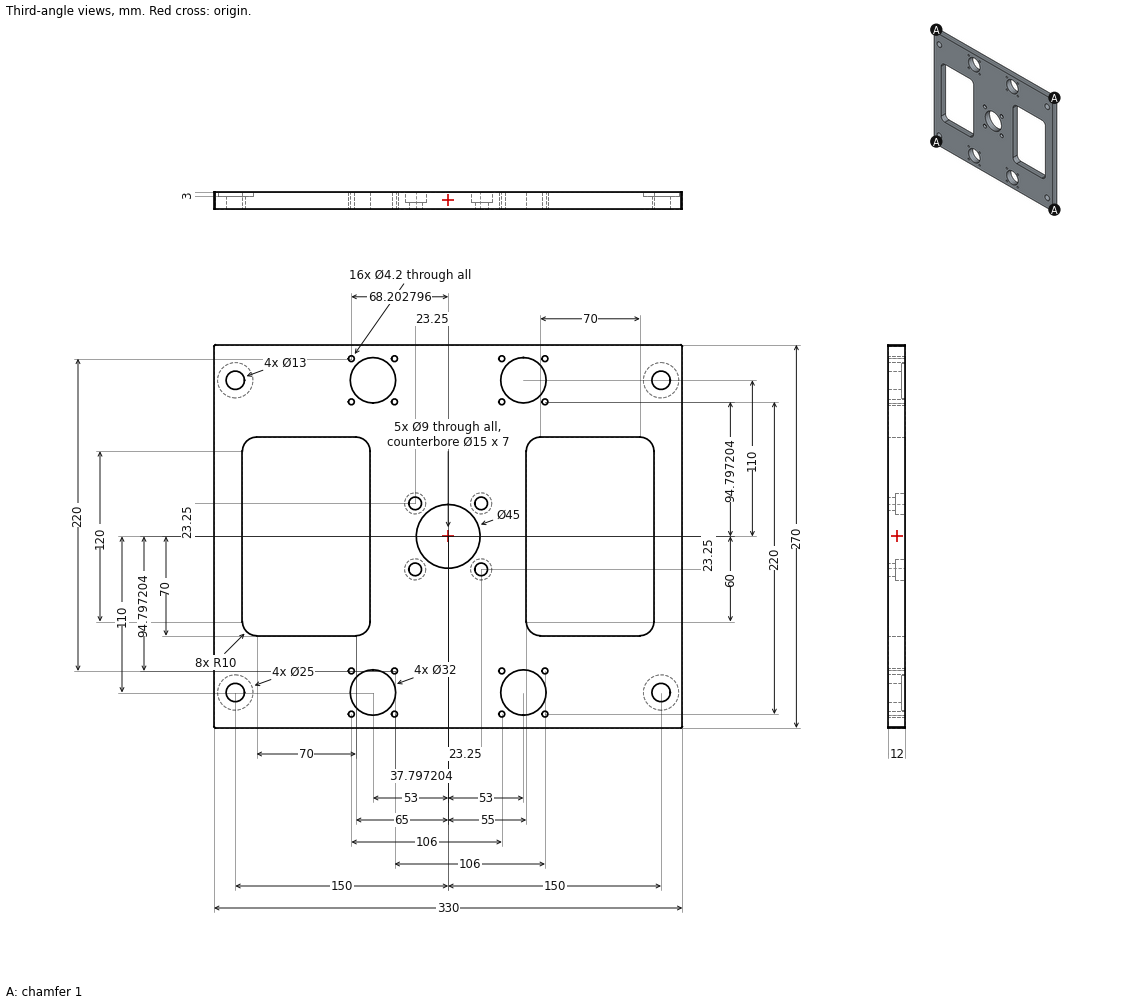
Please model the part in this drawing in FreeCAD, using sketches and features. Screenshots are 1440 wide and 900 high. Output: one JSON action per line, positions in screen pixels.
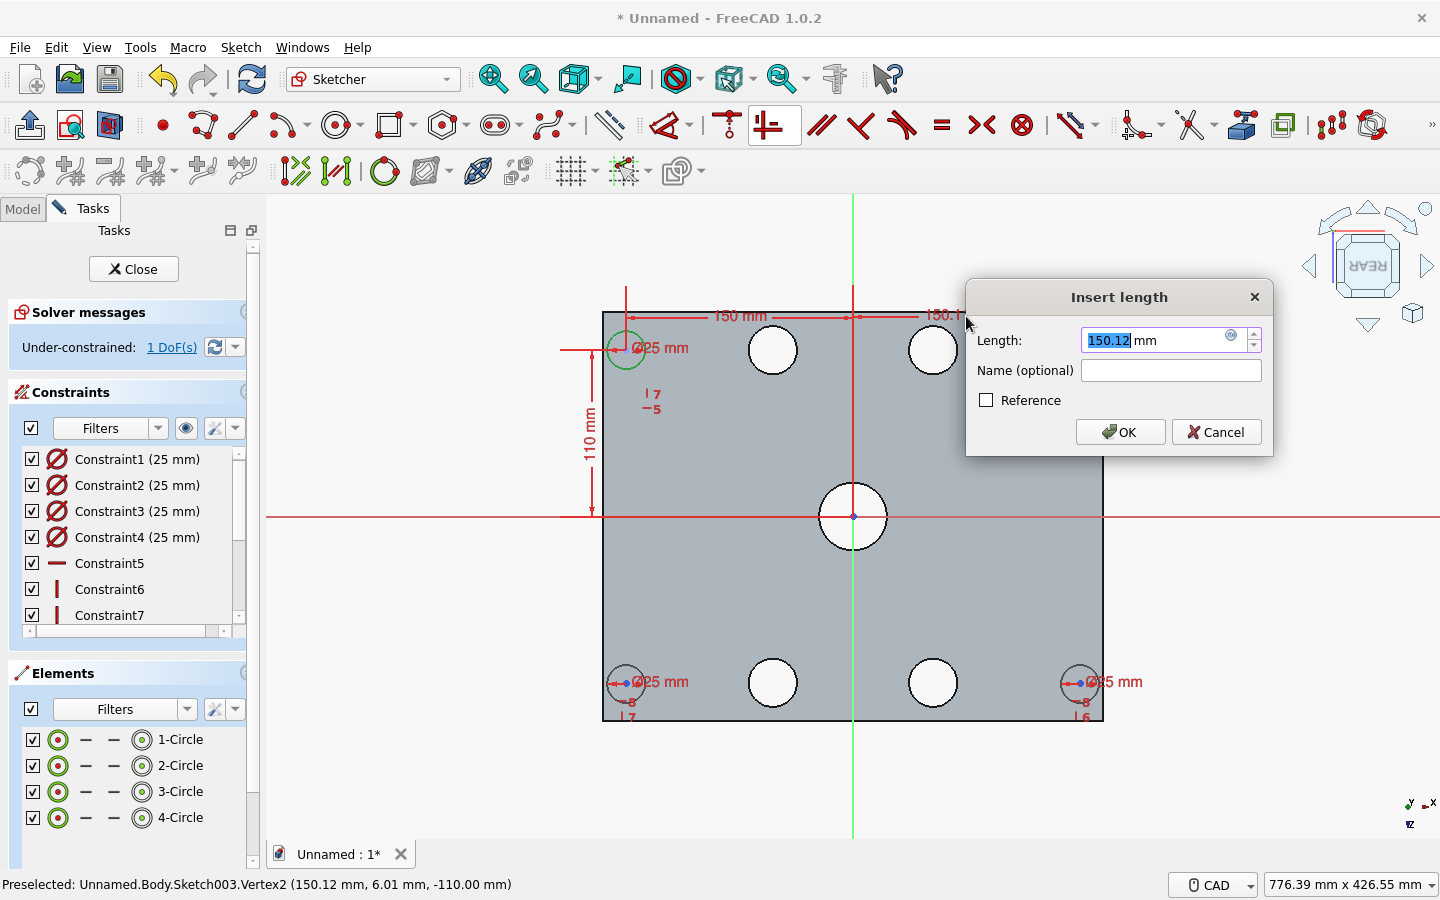
{"action": "type", "text": "150"}
{"action": "key", "text": "Return"}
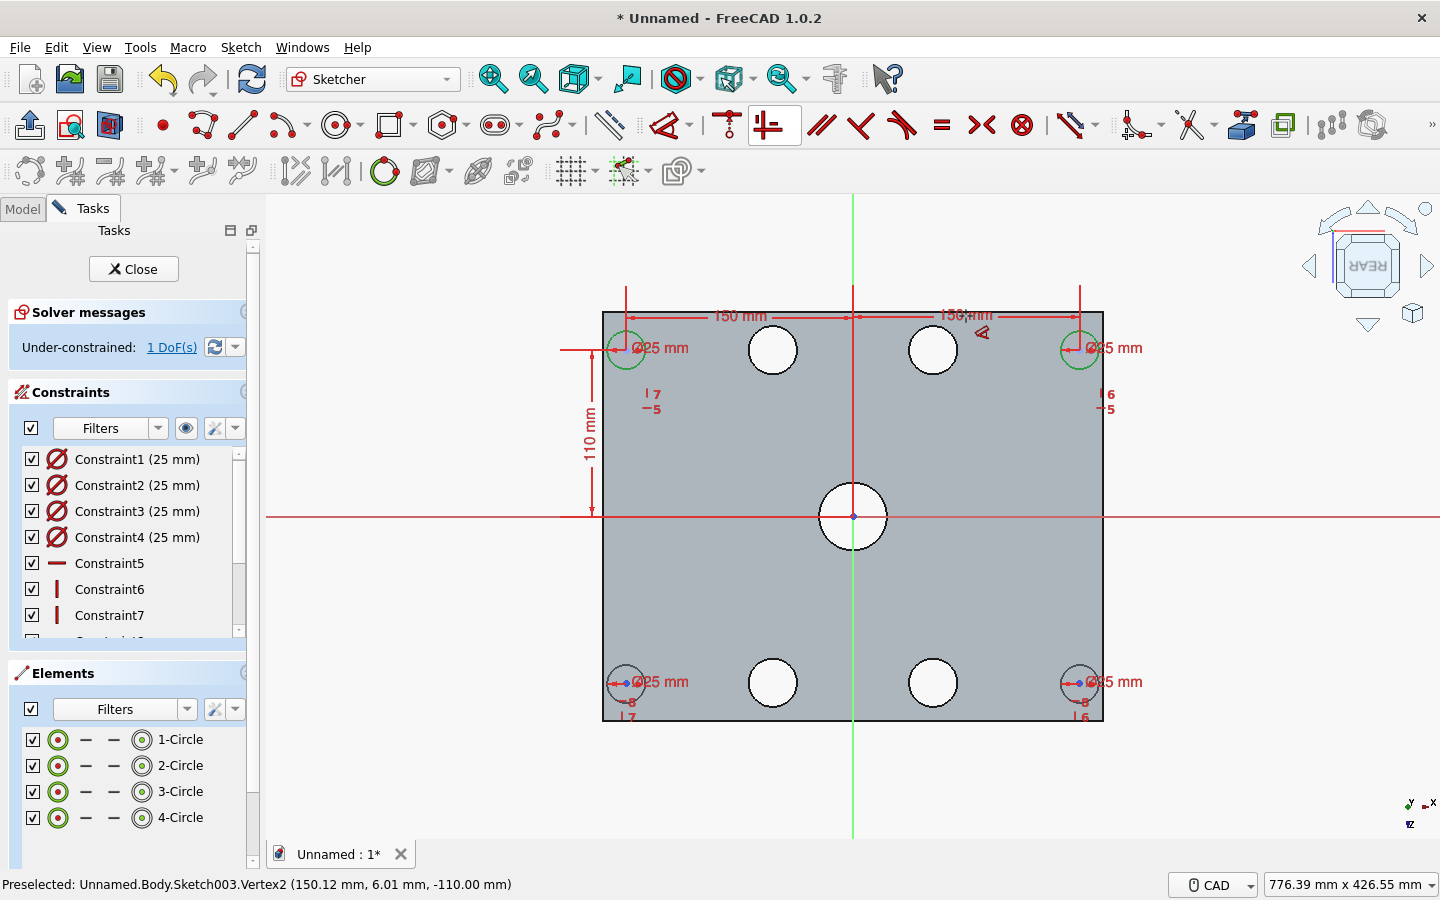
{"action": "left_click", "coordinate": [1080, 684]}
{"action": "left_click", "coordinate": [1114, 600]}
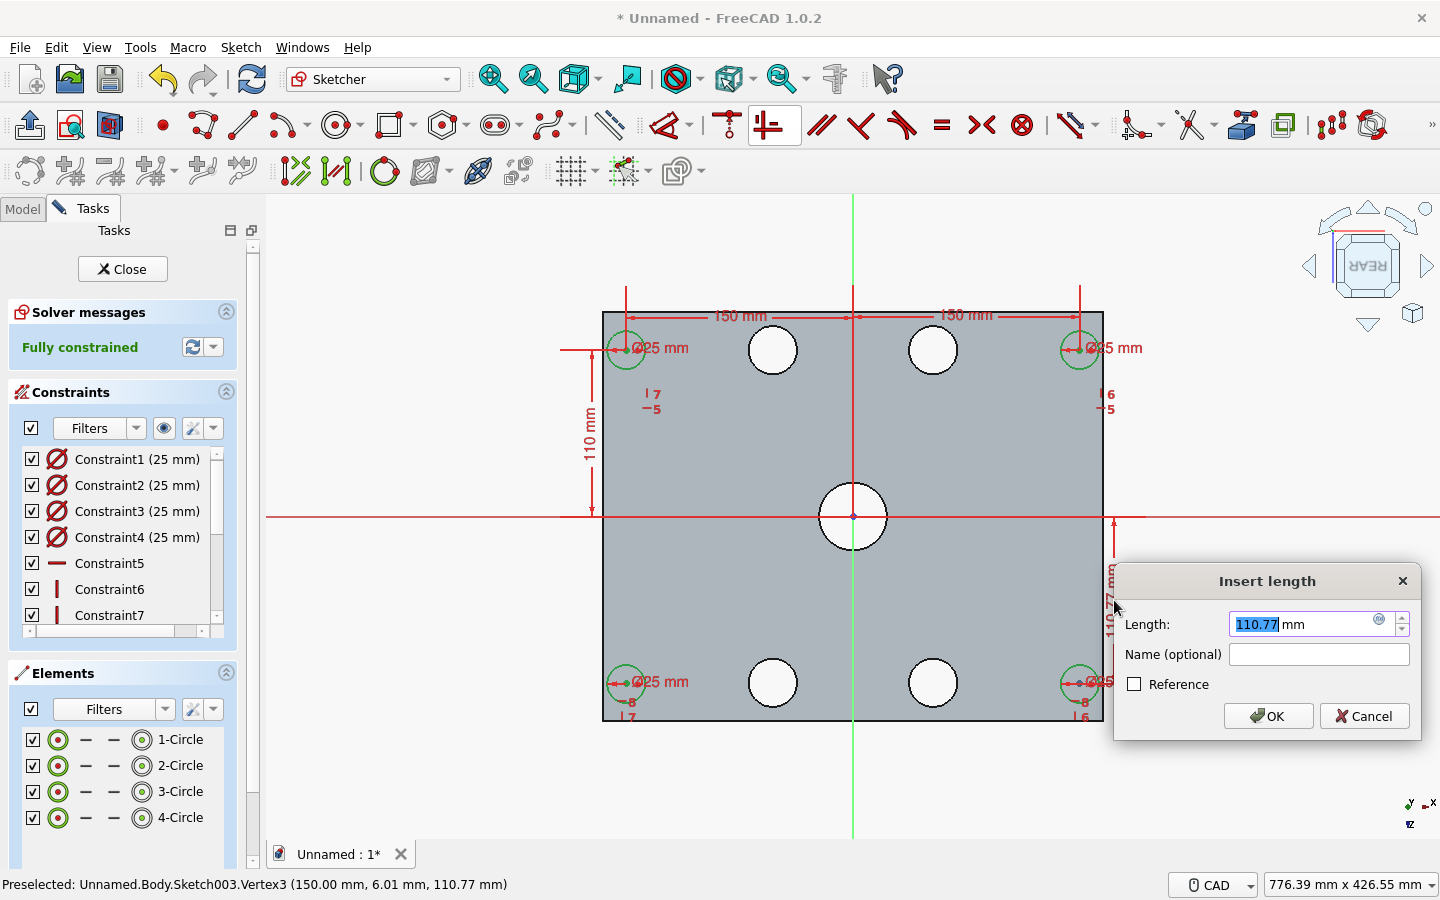
{"action": "type", "text": "110"}
{"action": "key", "text": "Return"}
{"action": "key", "text": "Escape"}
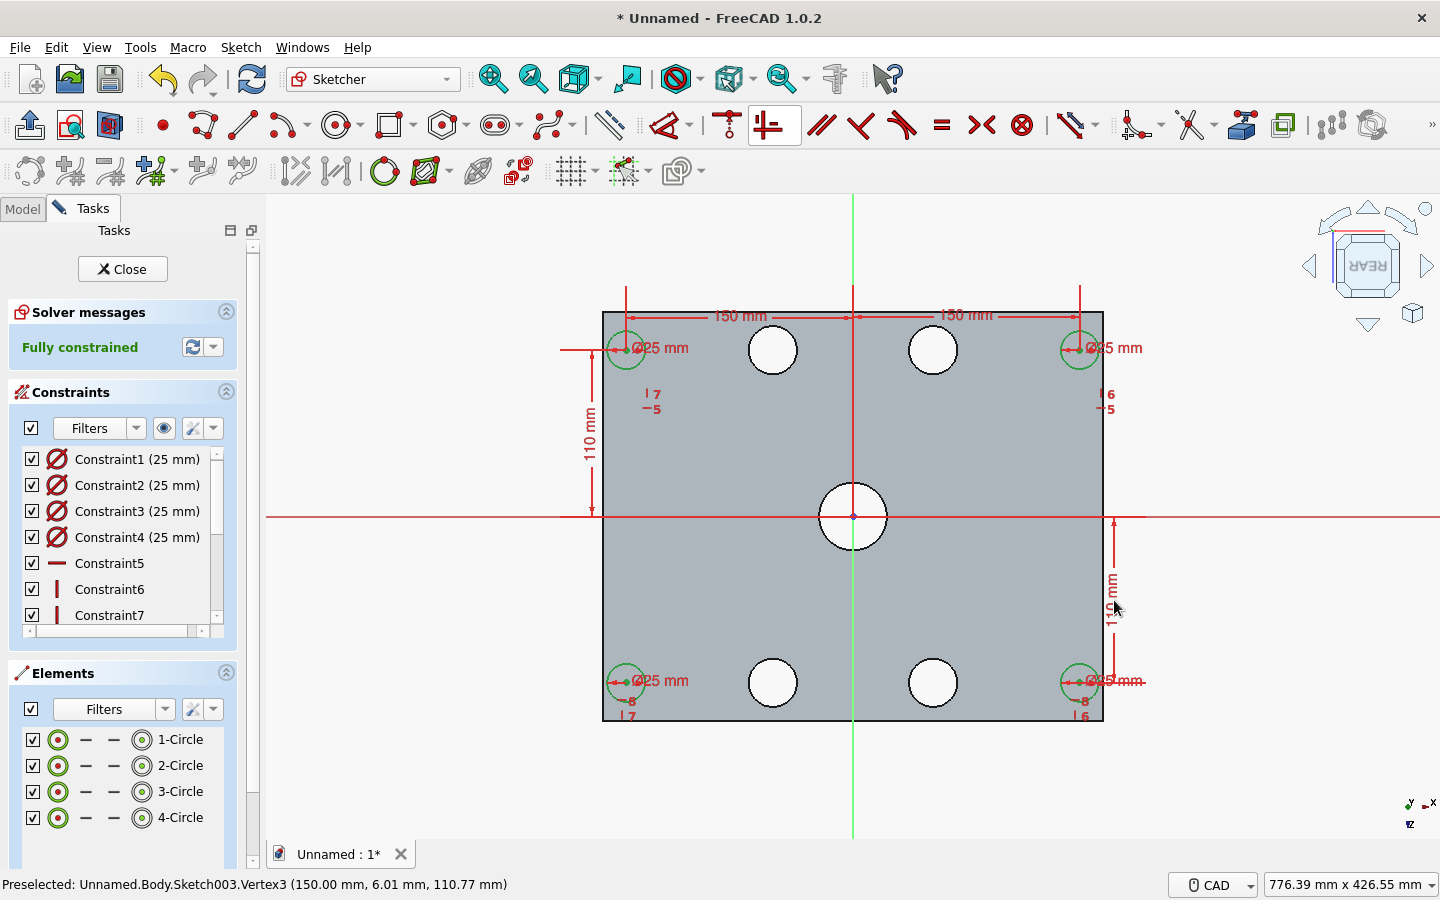
{"action": "left_click", "coordinate": [123, 269]}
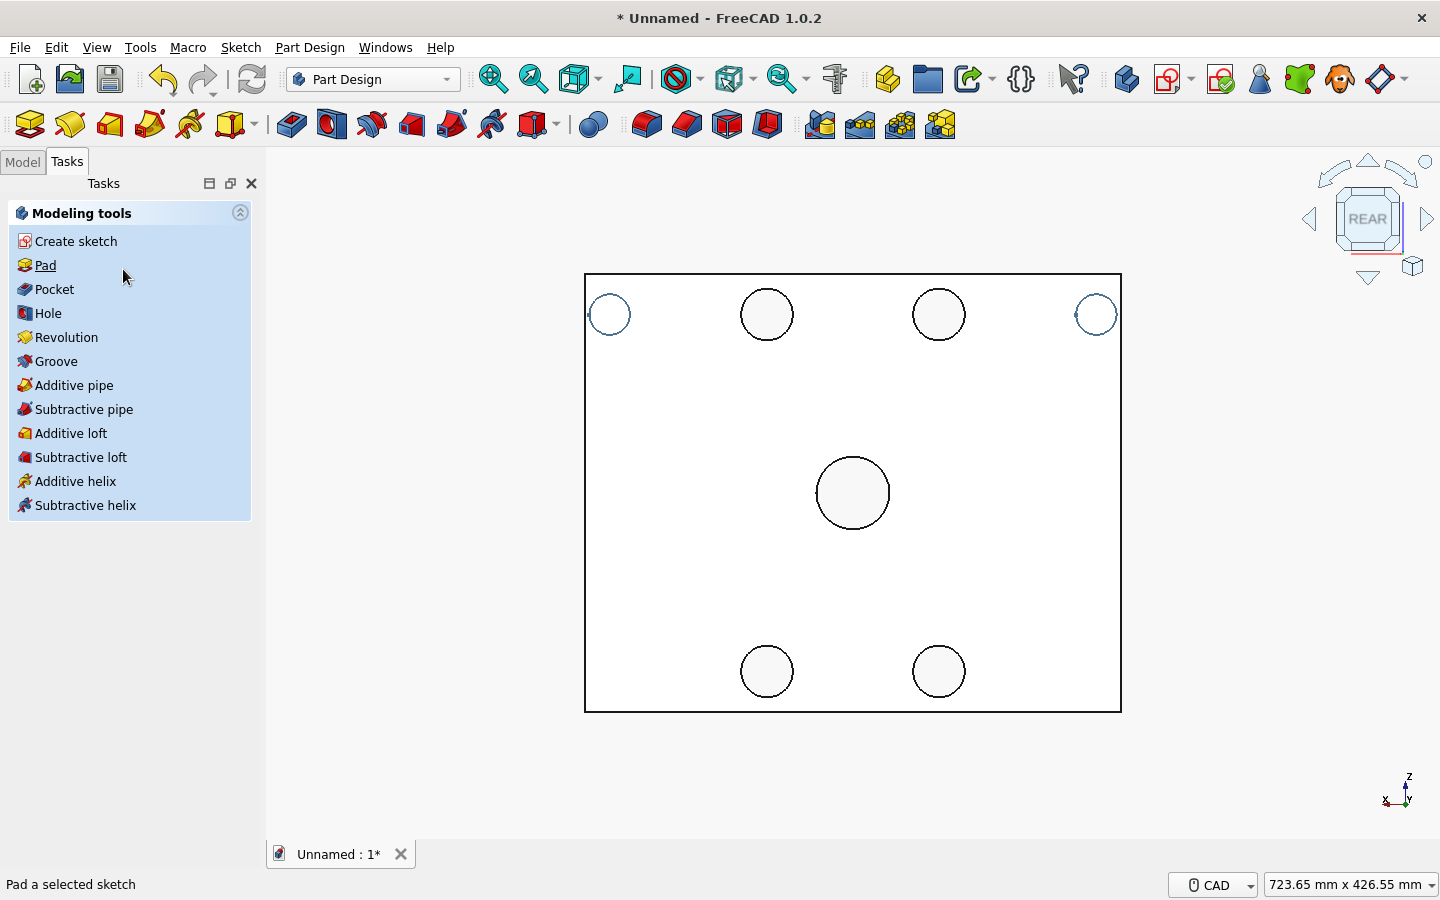
{"action": "left_click", "coordinate": [292, 124]}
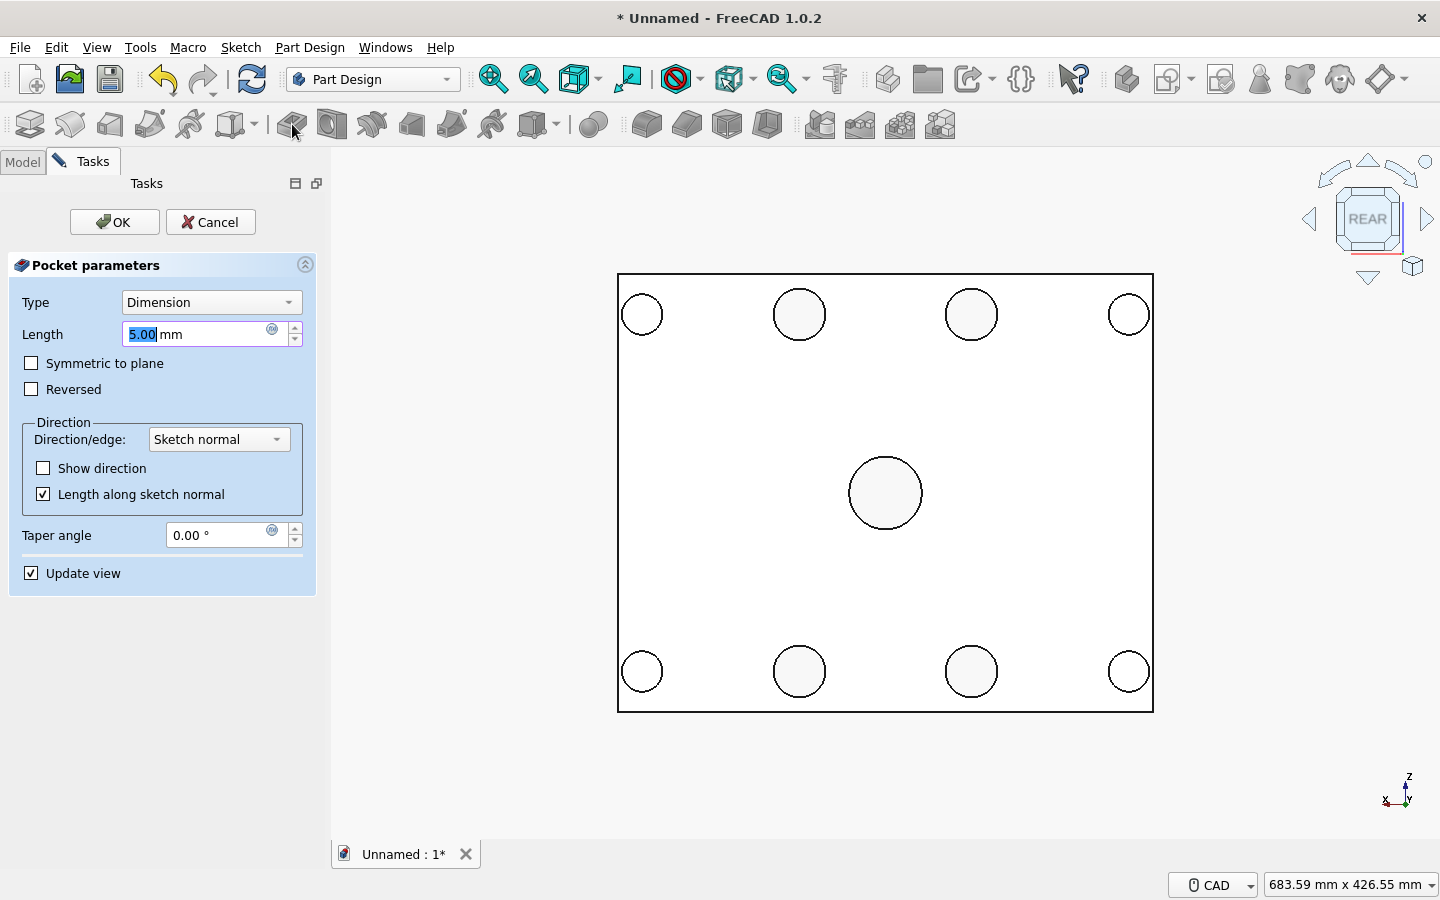
{"action": "type", "text": "3"}
{"action": "key", "text": "Tab"}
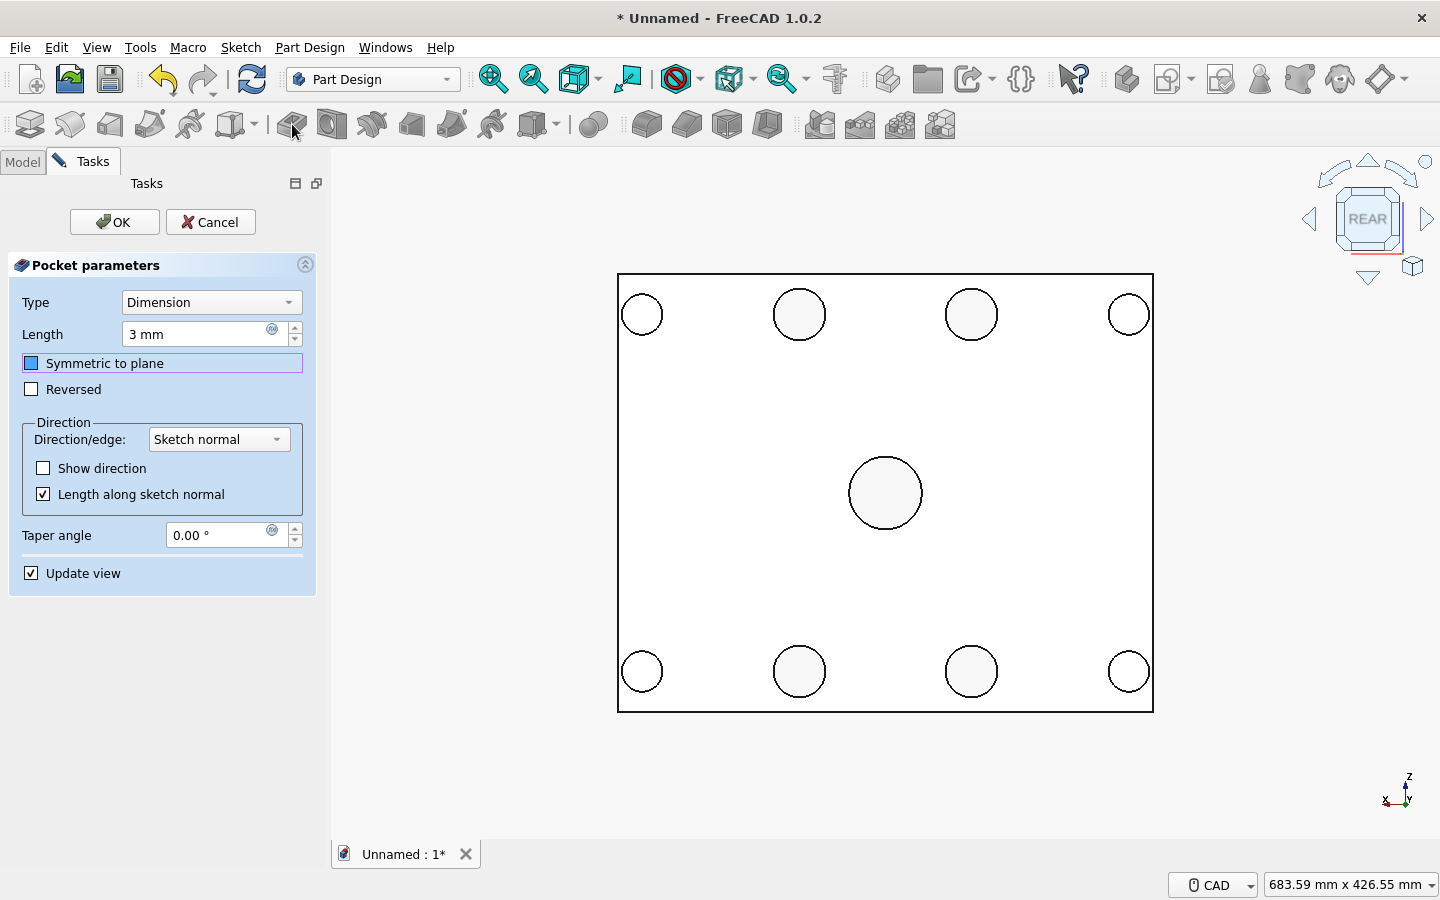
{"action": "left_click", "coordinate": [115, 222]}